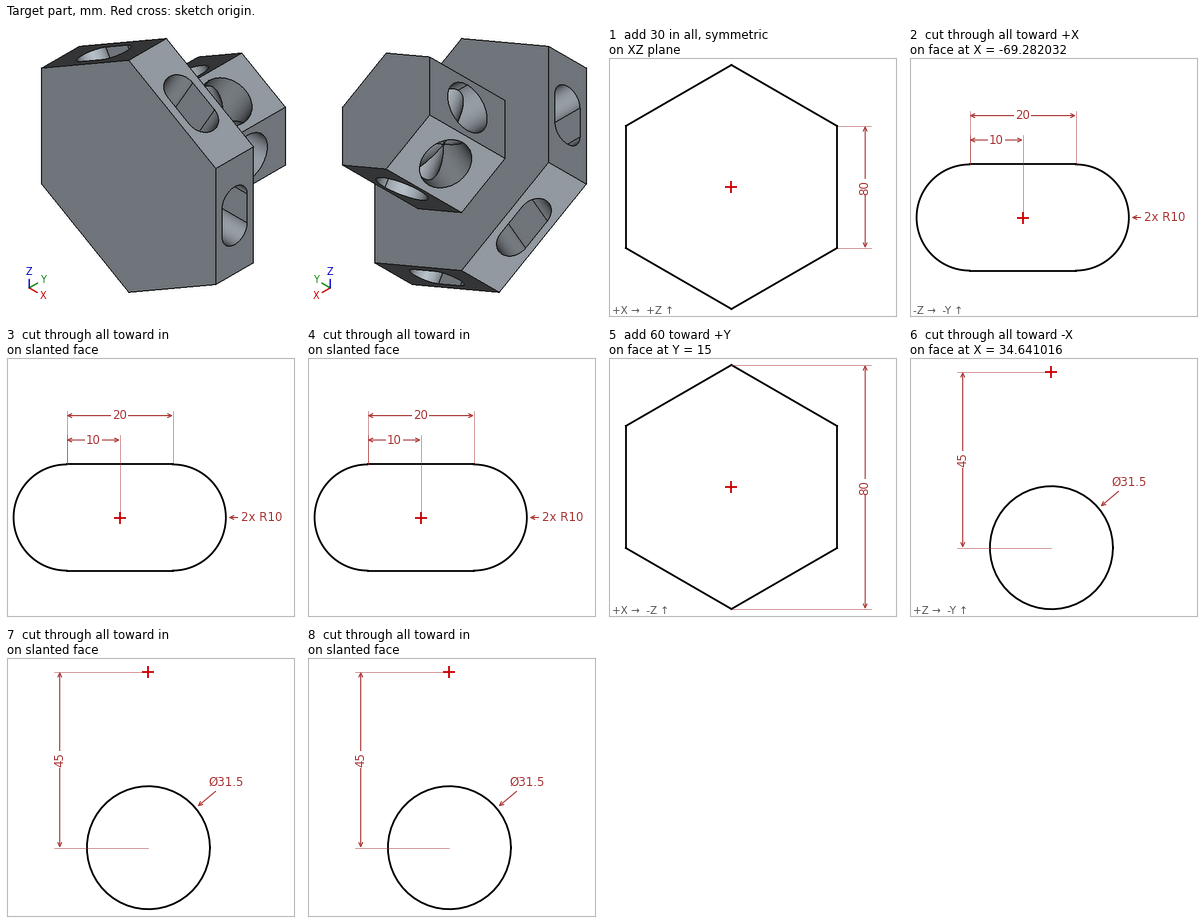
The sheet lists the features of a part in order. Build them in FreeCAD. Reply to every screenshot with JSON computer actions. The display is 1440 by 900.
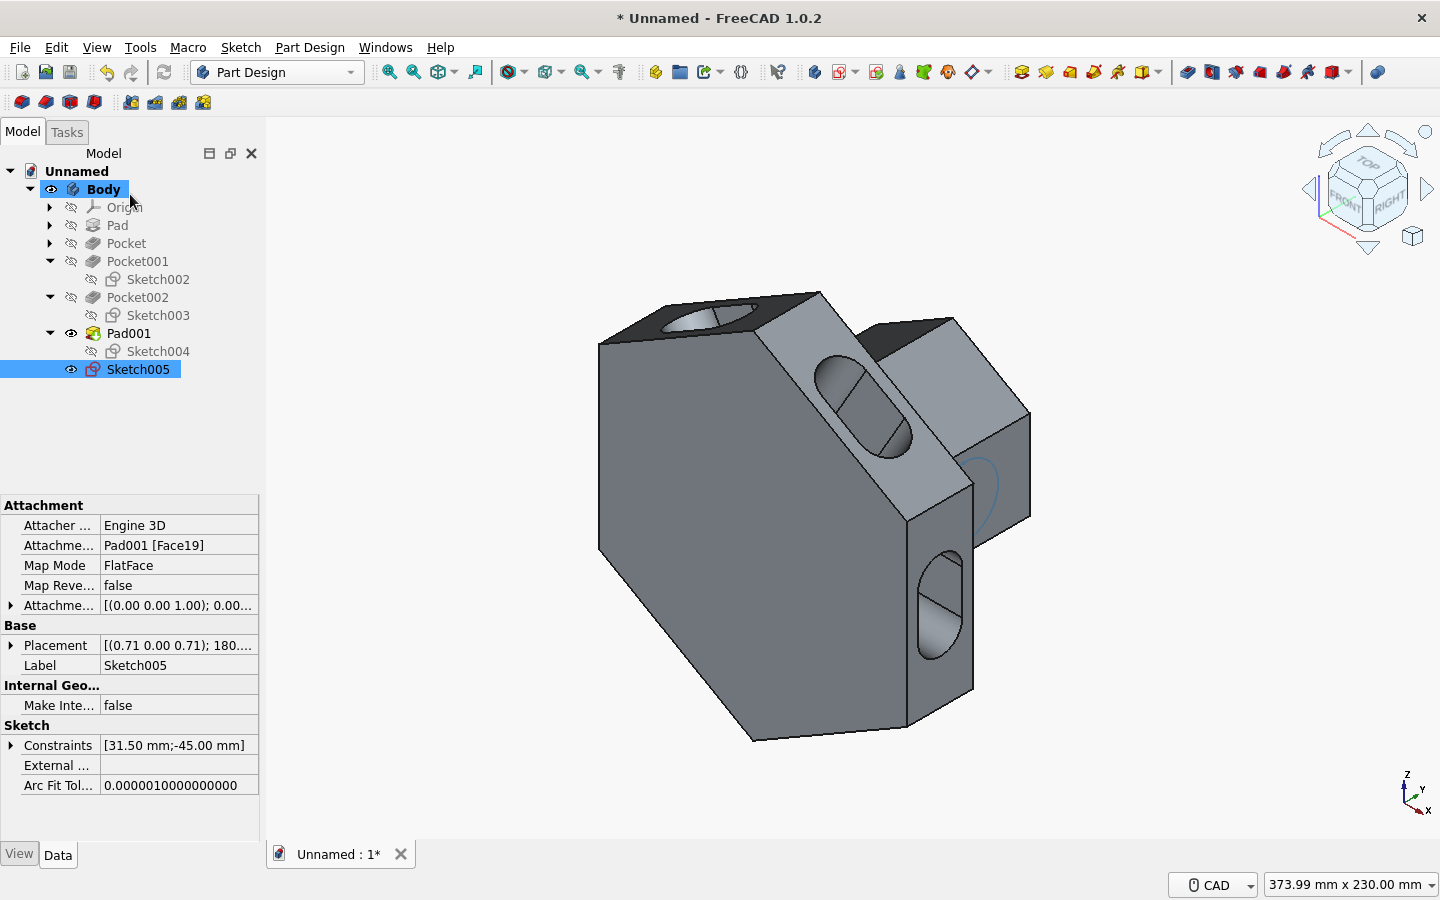
{"action": "left_click", "coordinate": [1188, 72]}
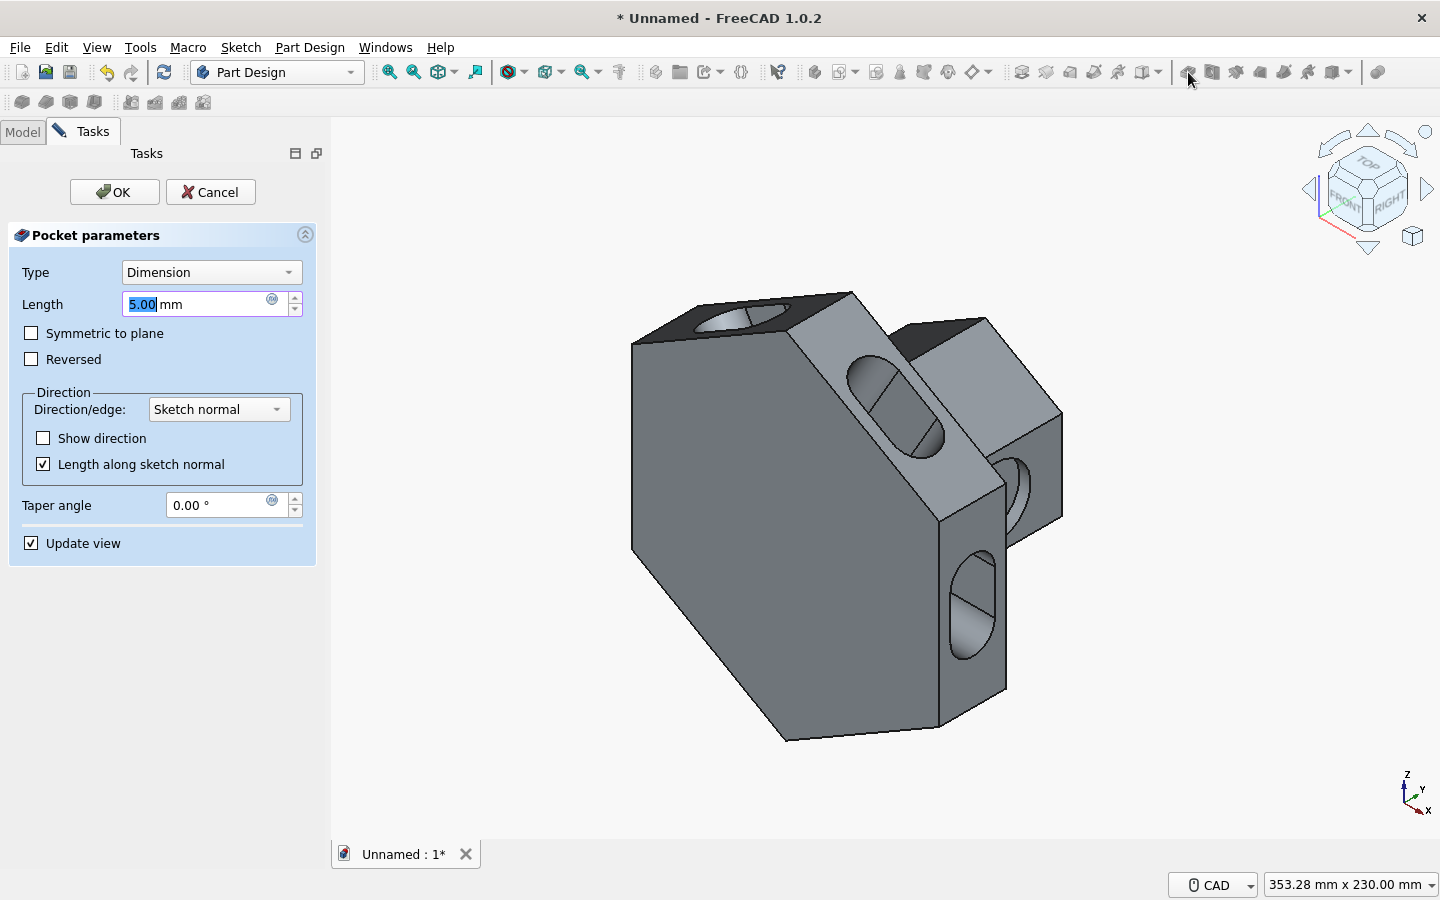
{"action": "left_click", "coordinate": [212, 272]}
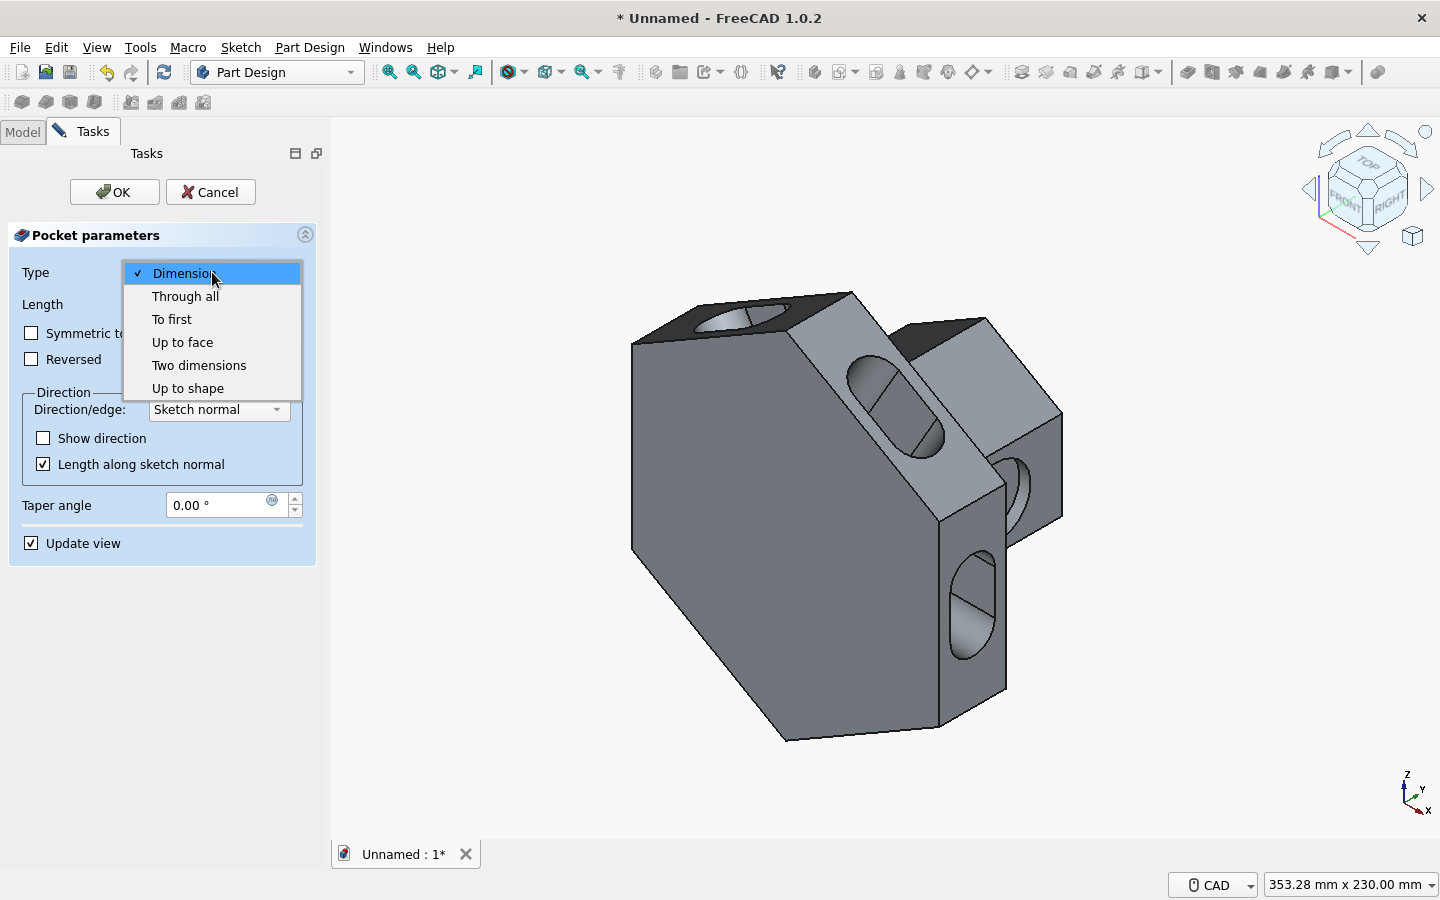
{"action": "left_click", "coordinate": [212, 296]}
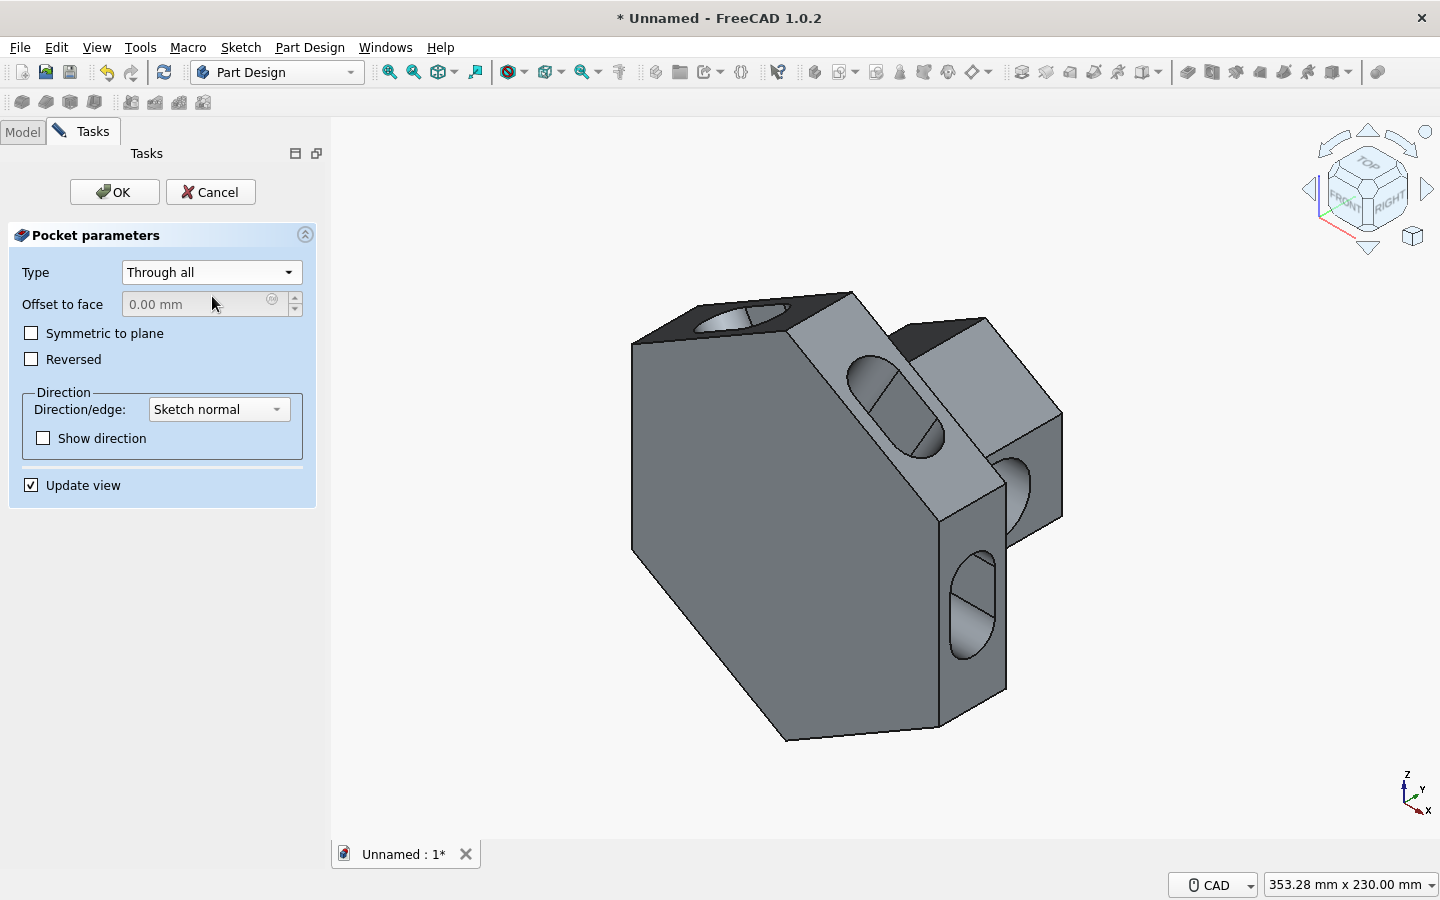
{"action": "left_click", "coordinate": [115, 192]}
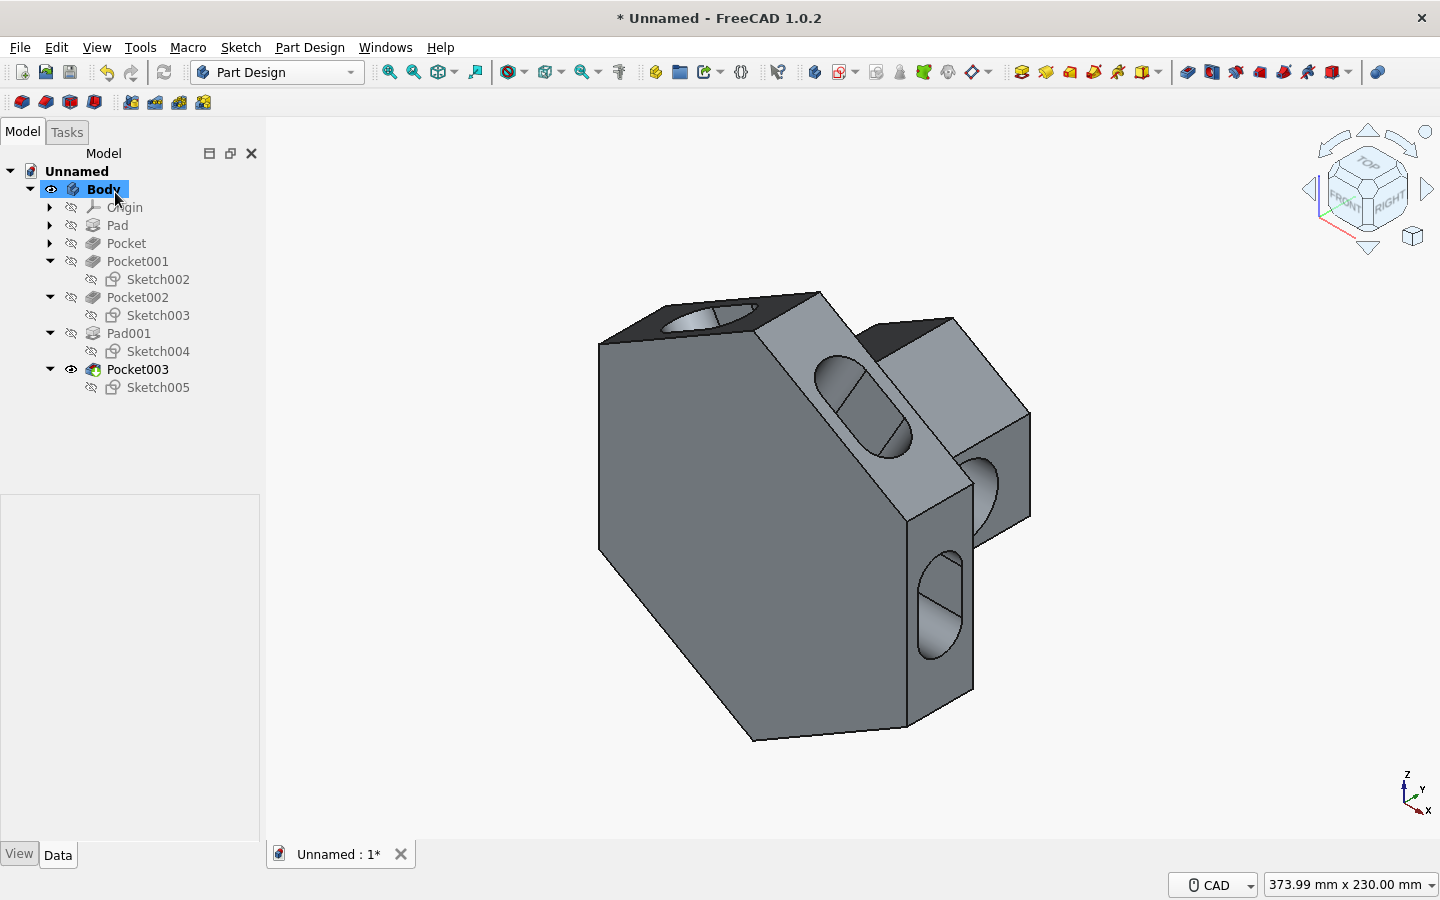
{"action": "key", "text": "5"}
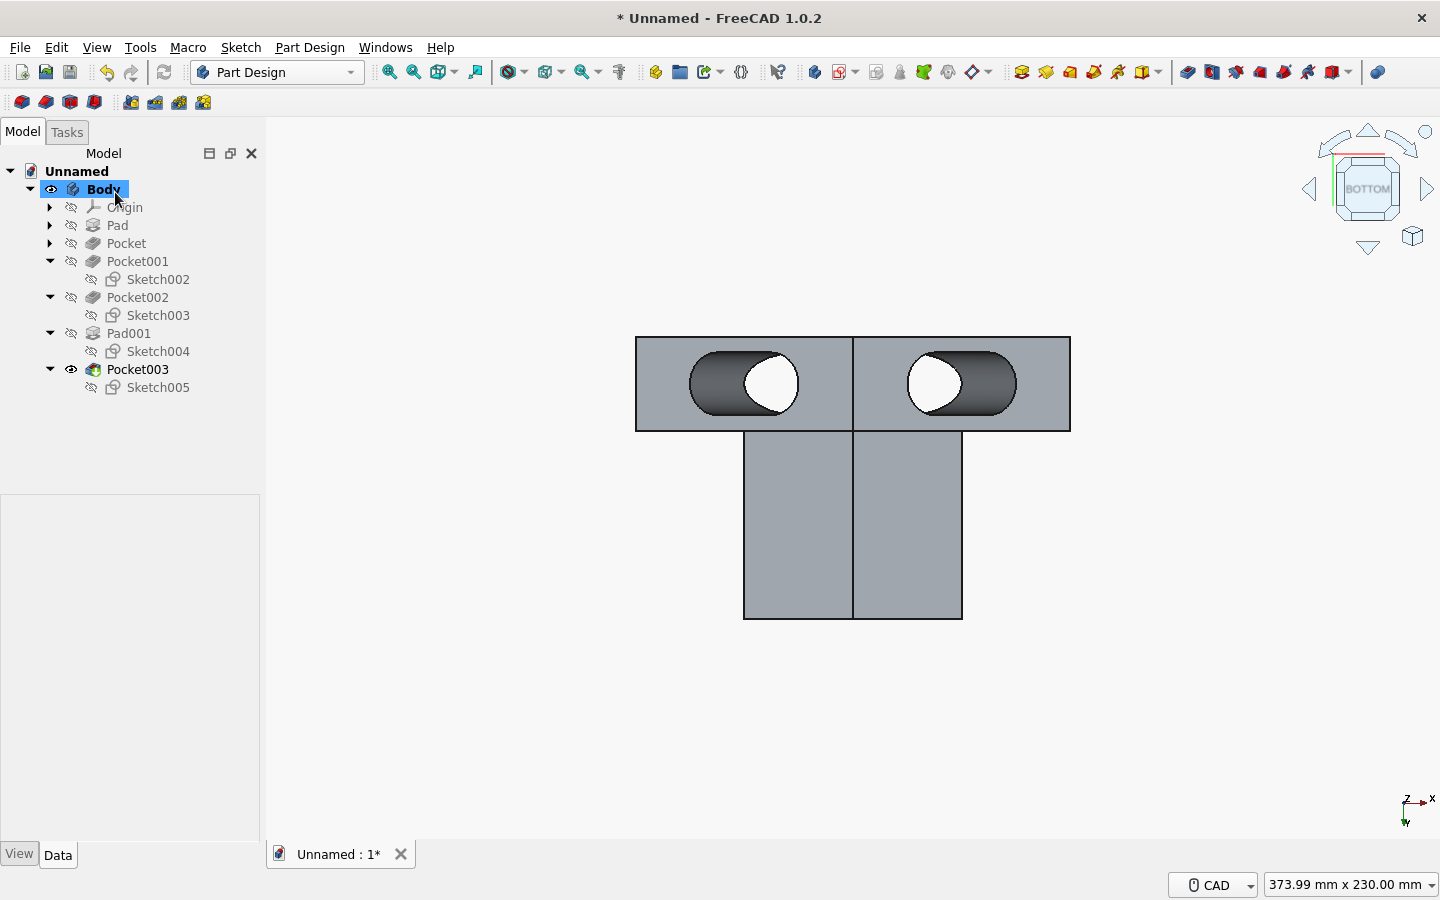
{"action": "left_click", "coordinate": [390, 72]}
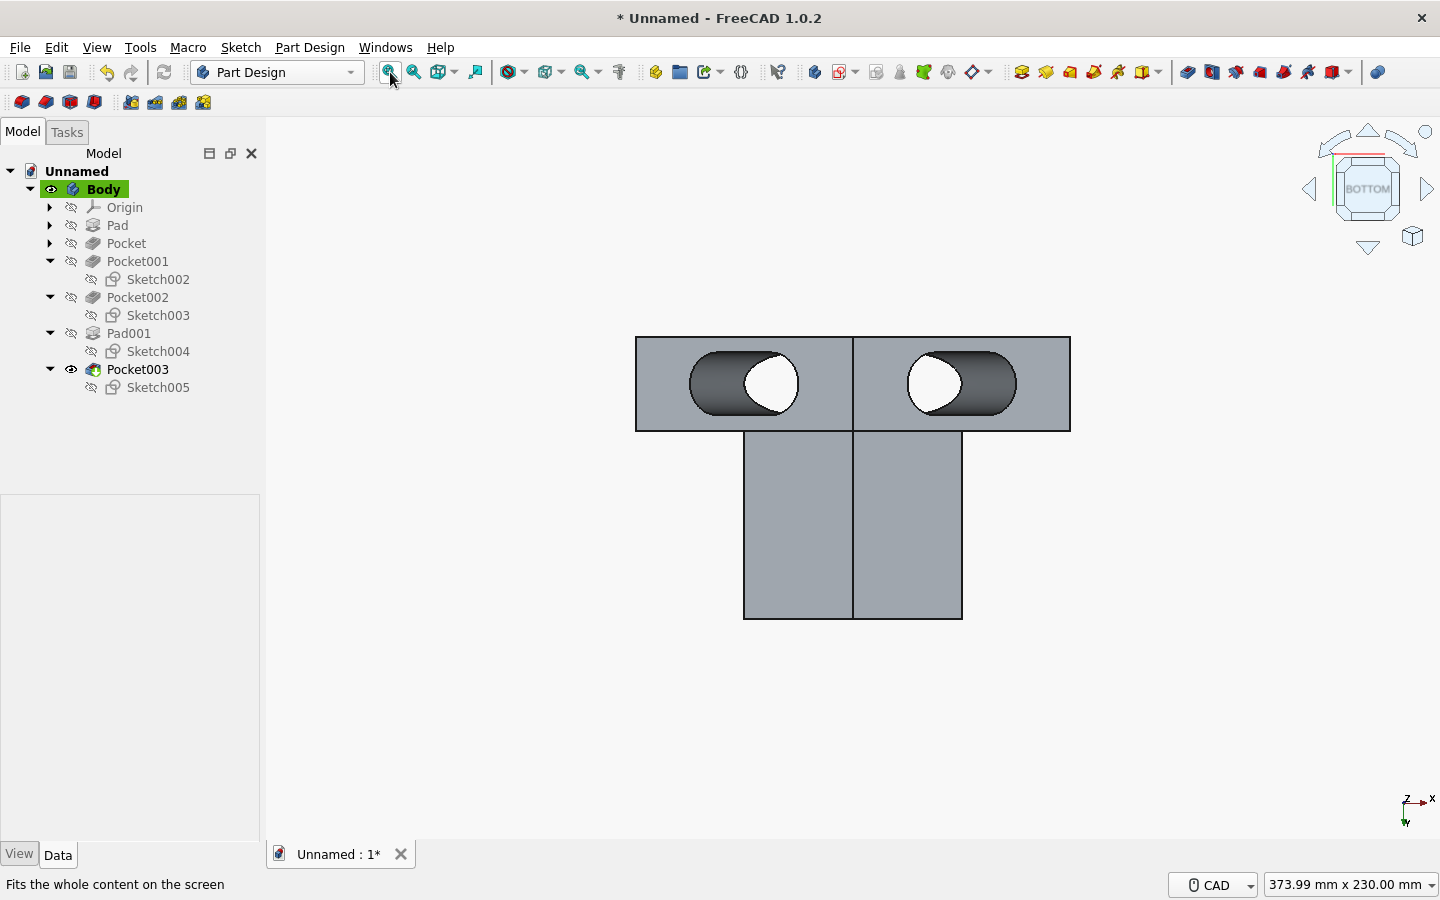
{"action": "left_click", "coordinate": [907, 551]}